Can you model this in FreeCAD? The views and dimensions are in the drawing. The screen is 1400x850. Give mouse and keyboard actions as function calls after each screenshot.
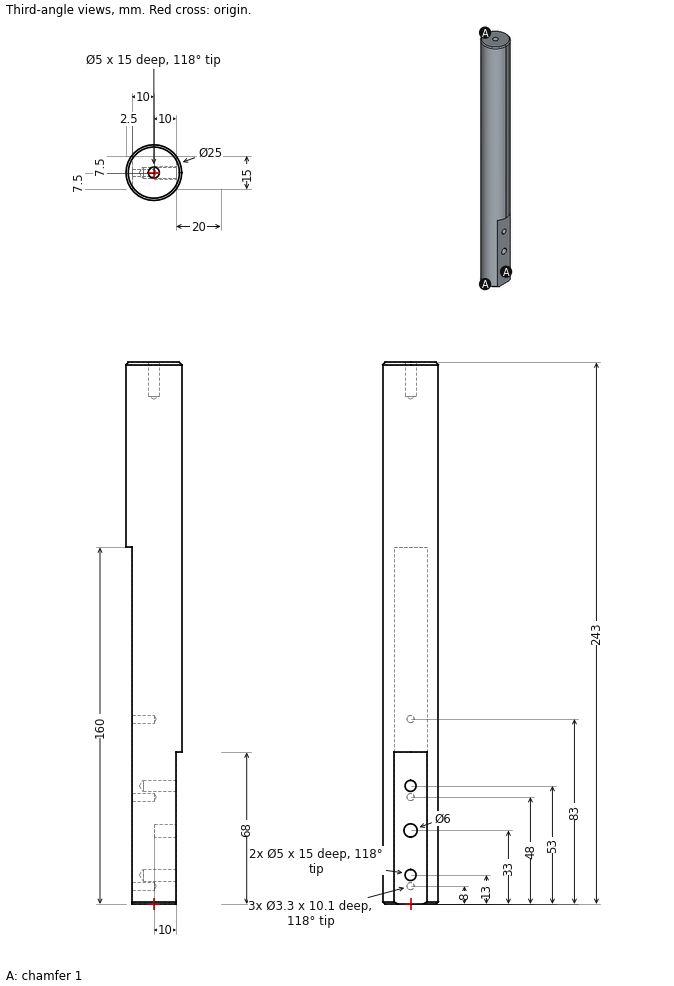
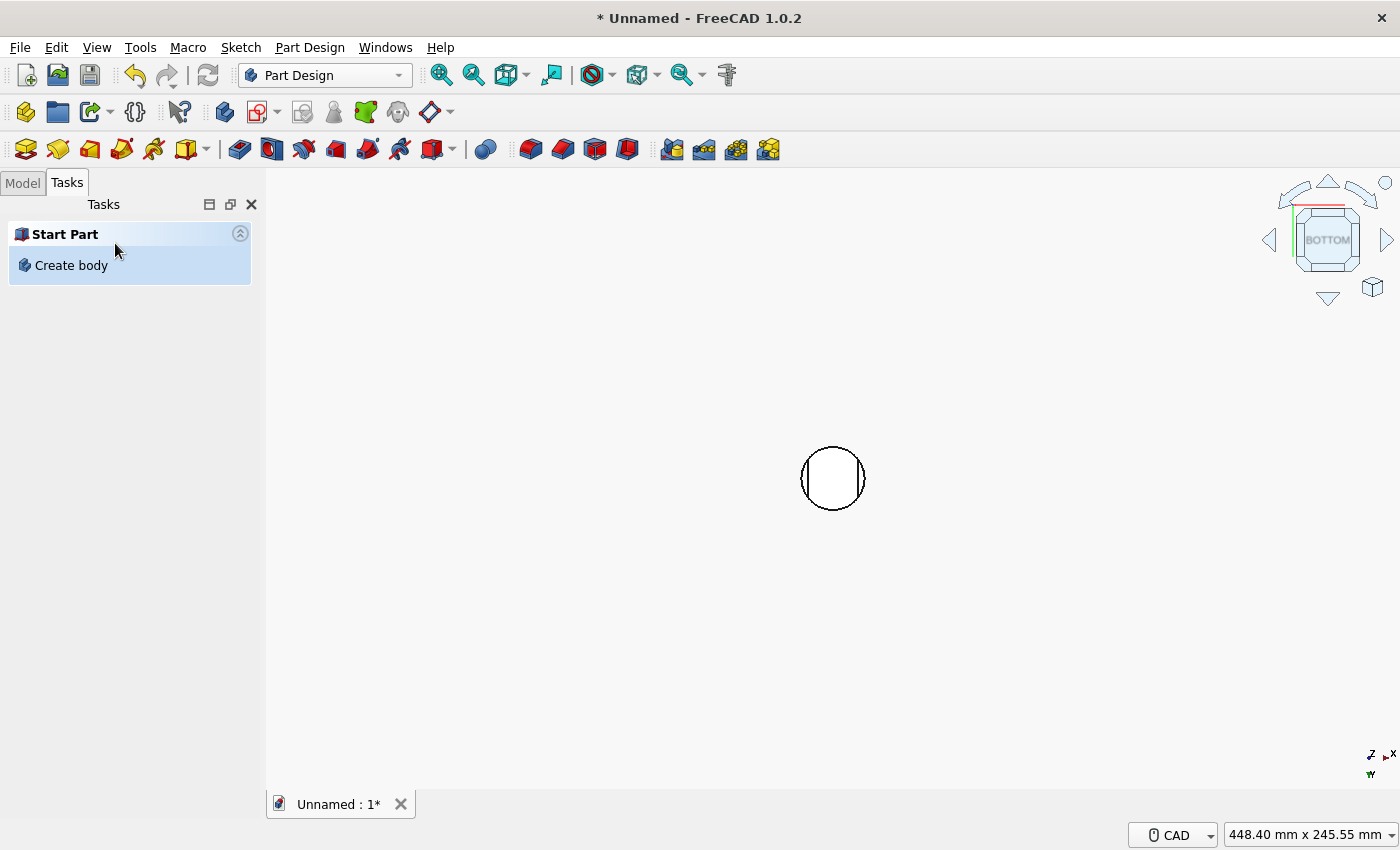
key(v)
key(f)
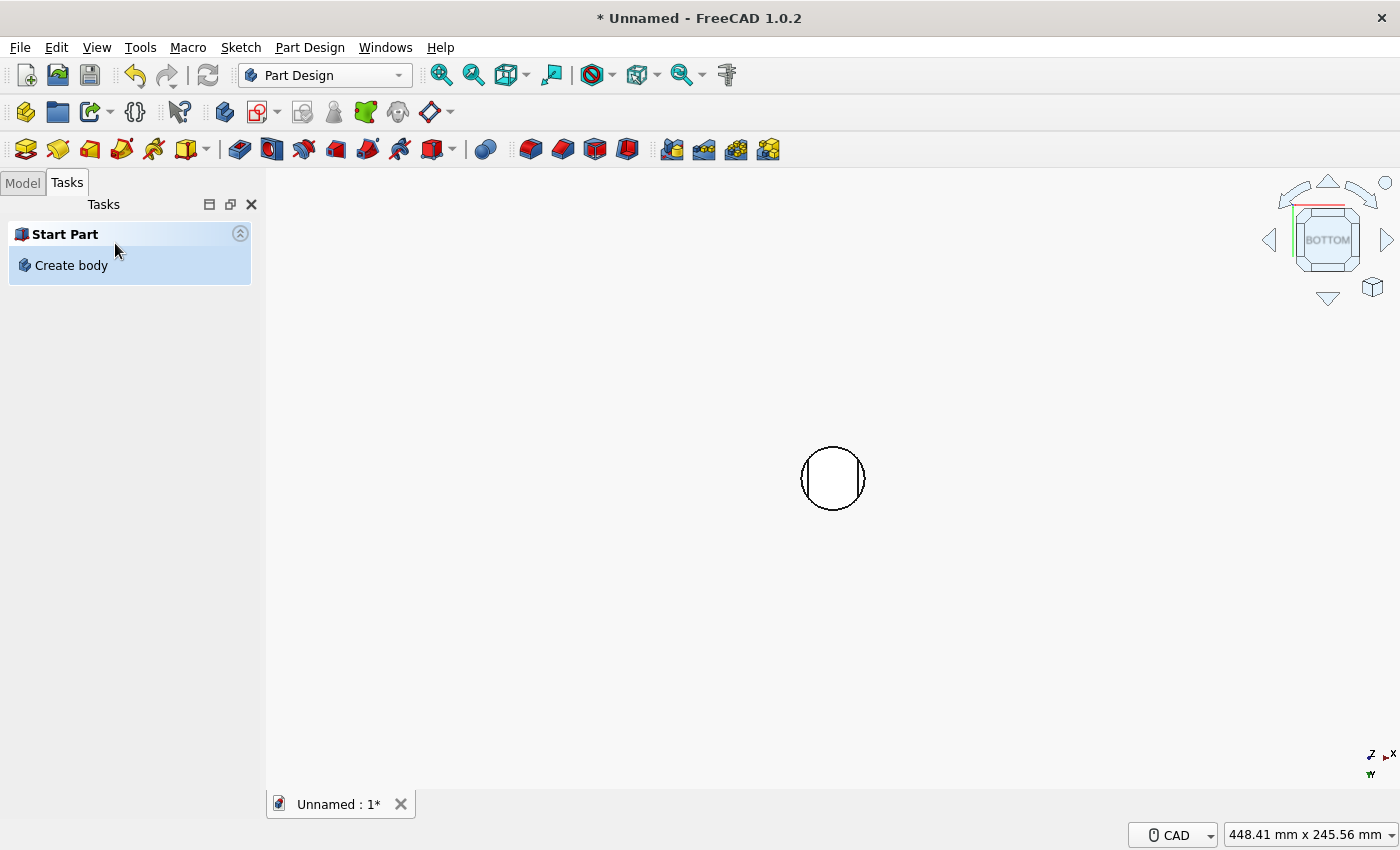
key(6)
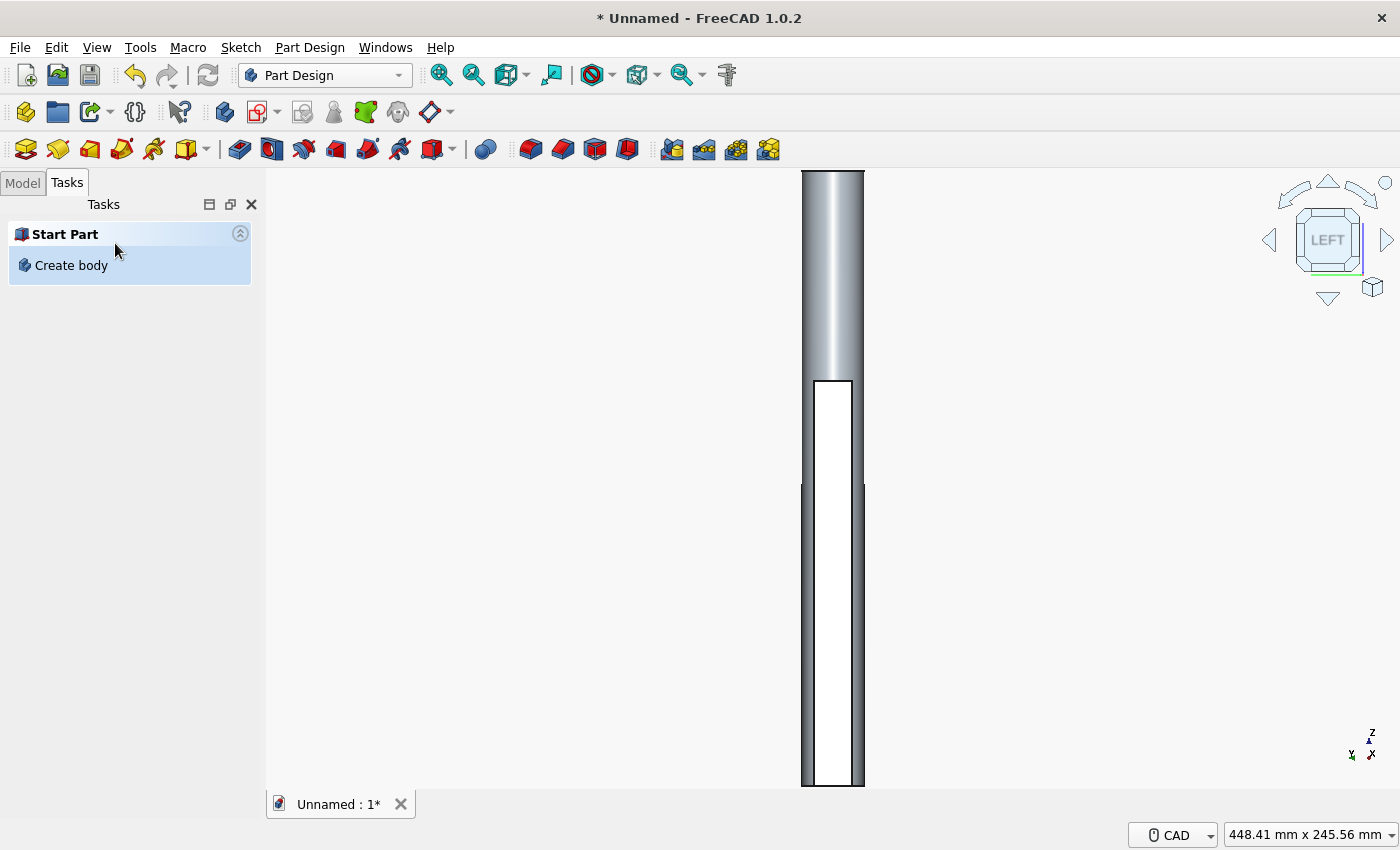
click(833, 409)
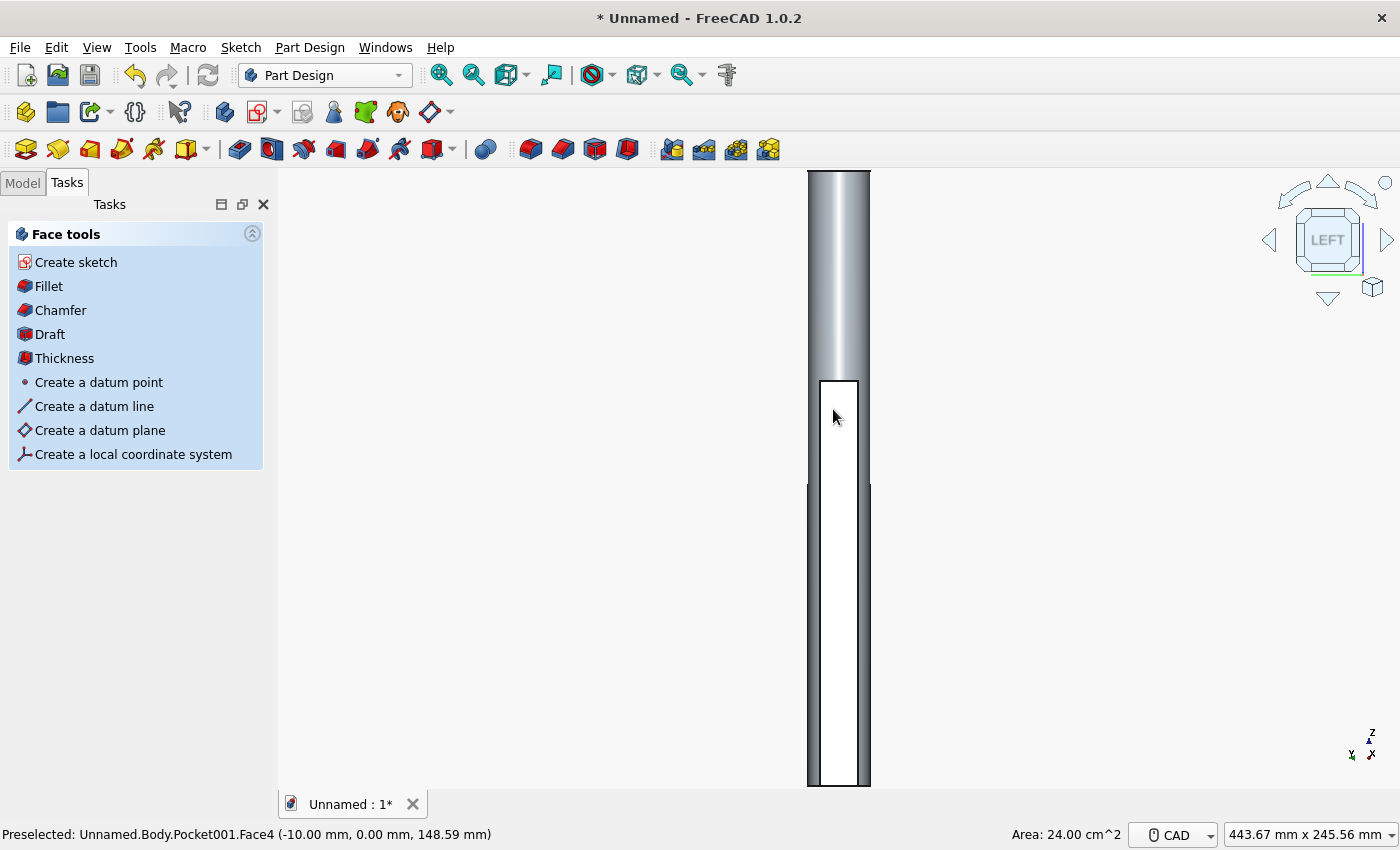
click(258, 112)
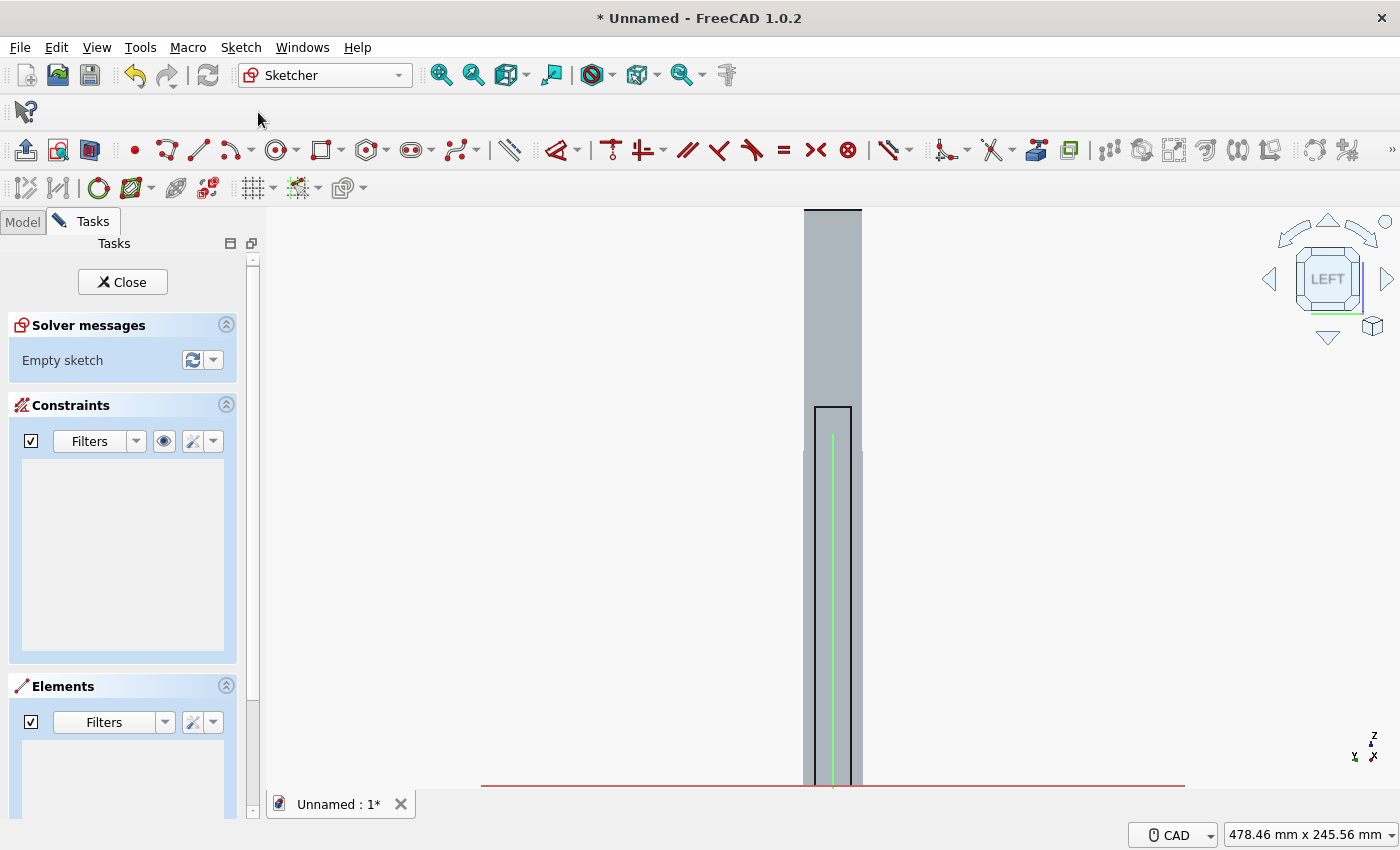
scroll(764, 498, down, 5)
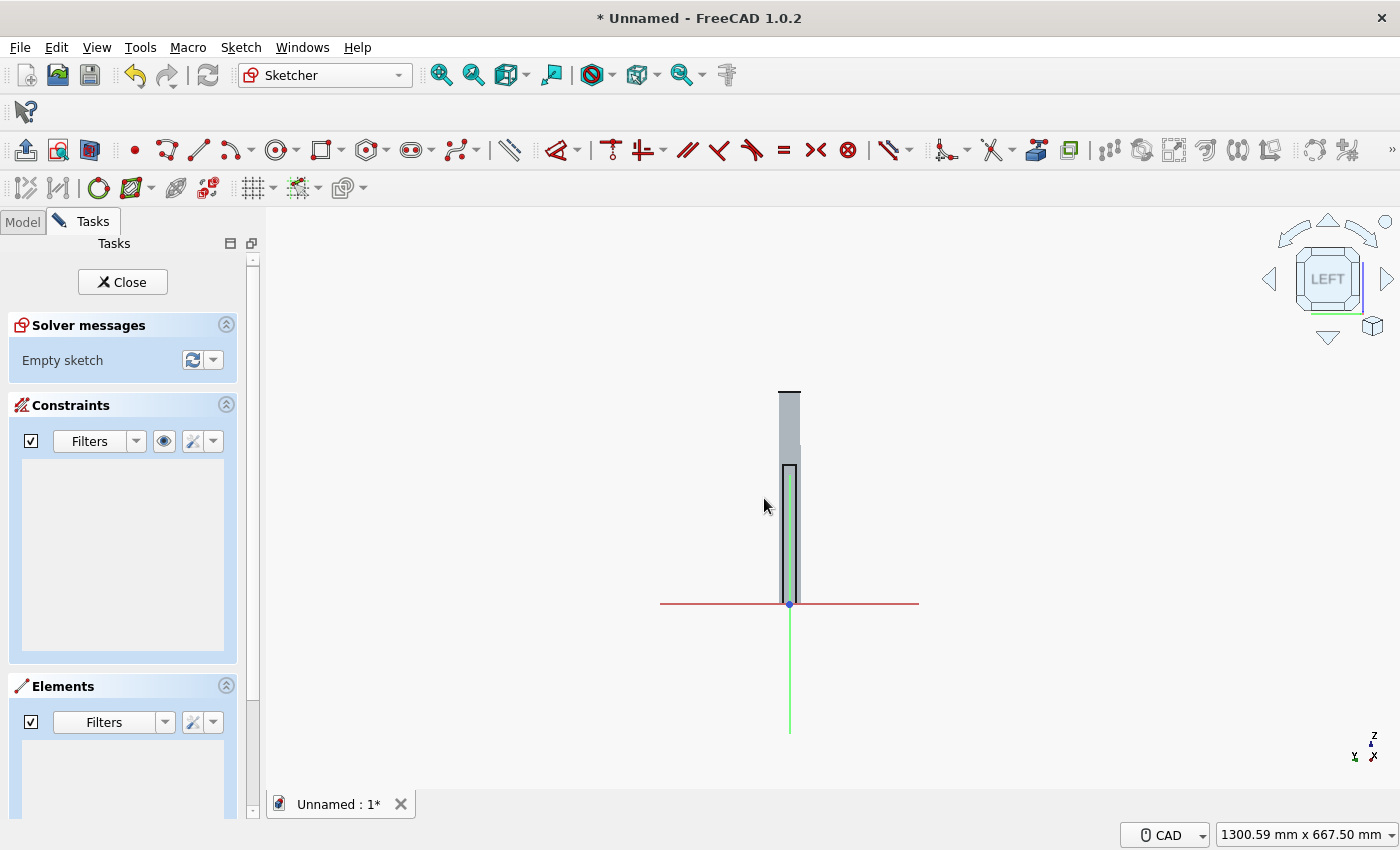
scroll(796, 585, up, 8)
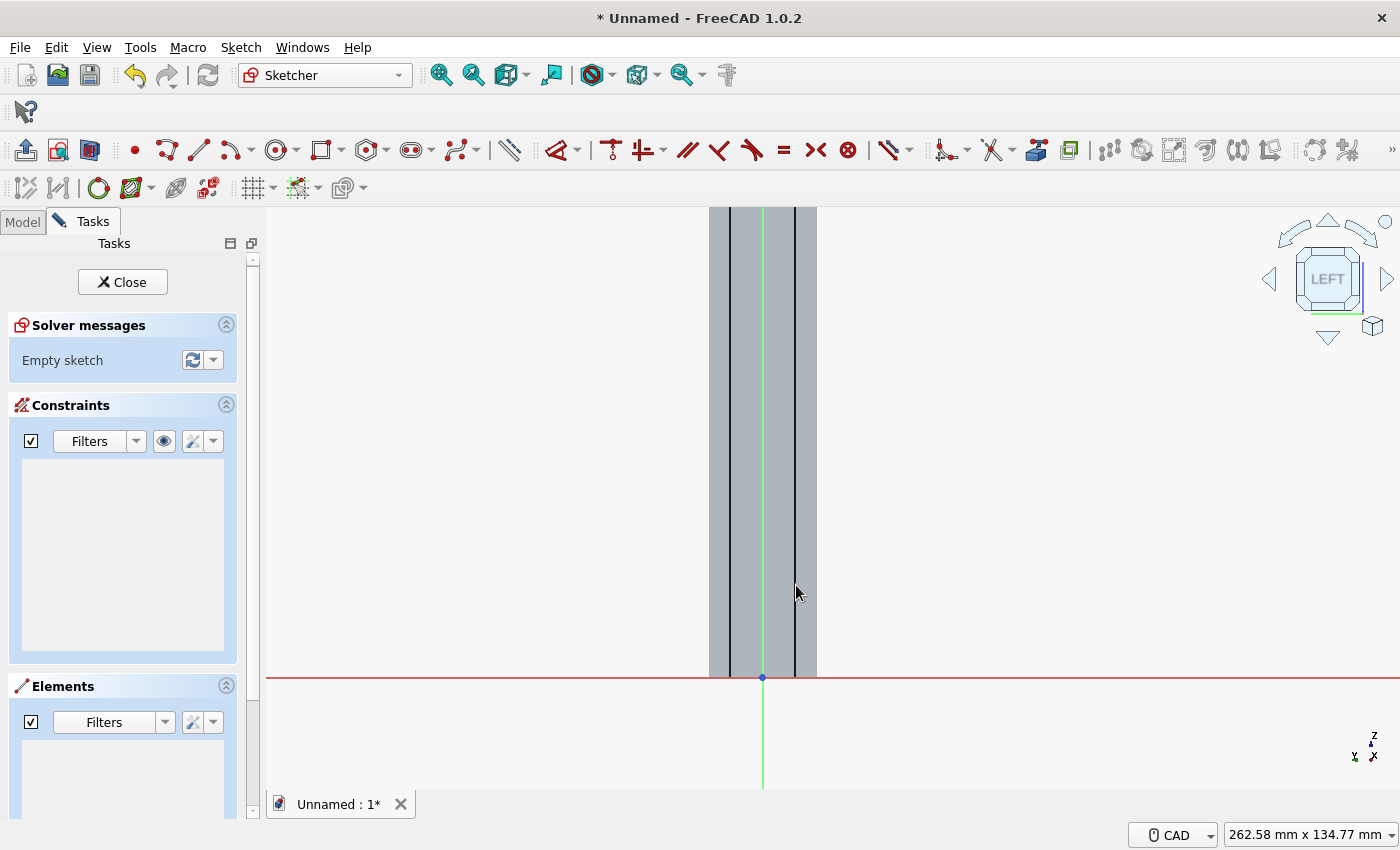
click(276, 150)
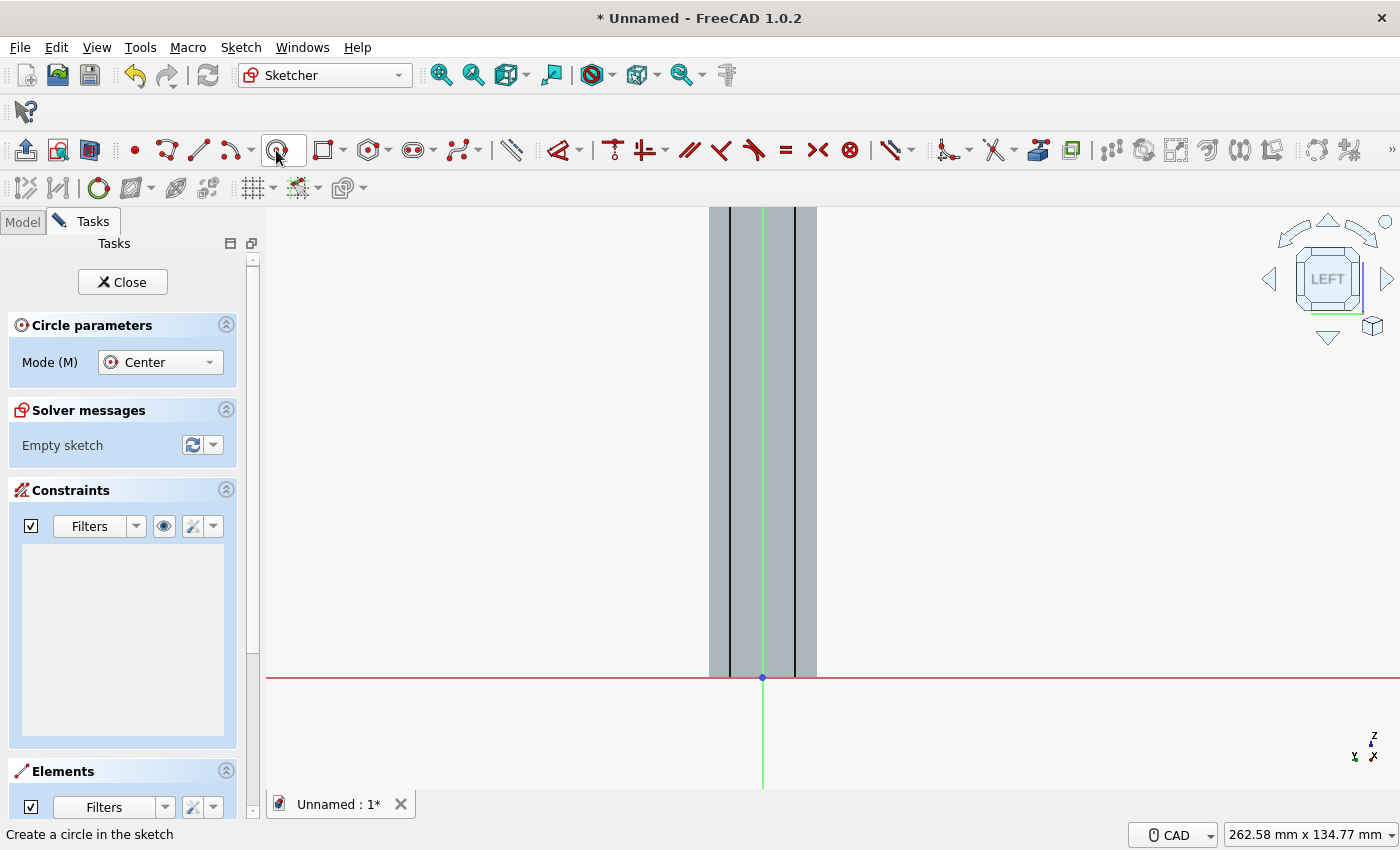
scroll(763, 643, up, 6)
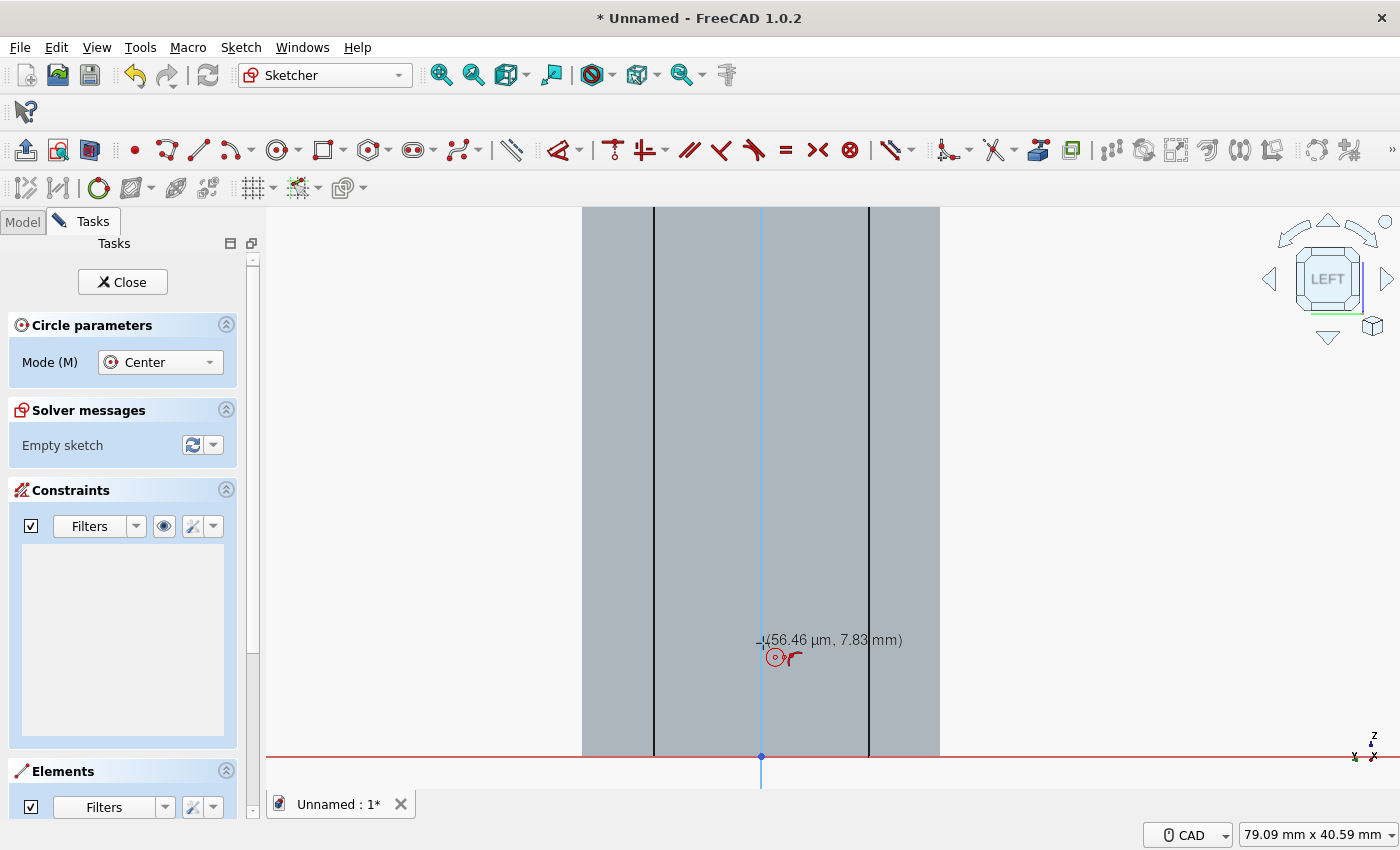
click(761, 642)
click(778, 625)